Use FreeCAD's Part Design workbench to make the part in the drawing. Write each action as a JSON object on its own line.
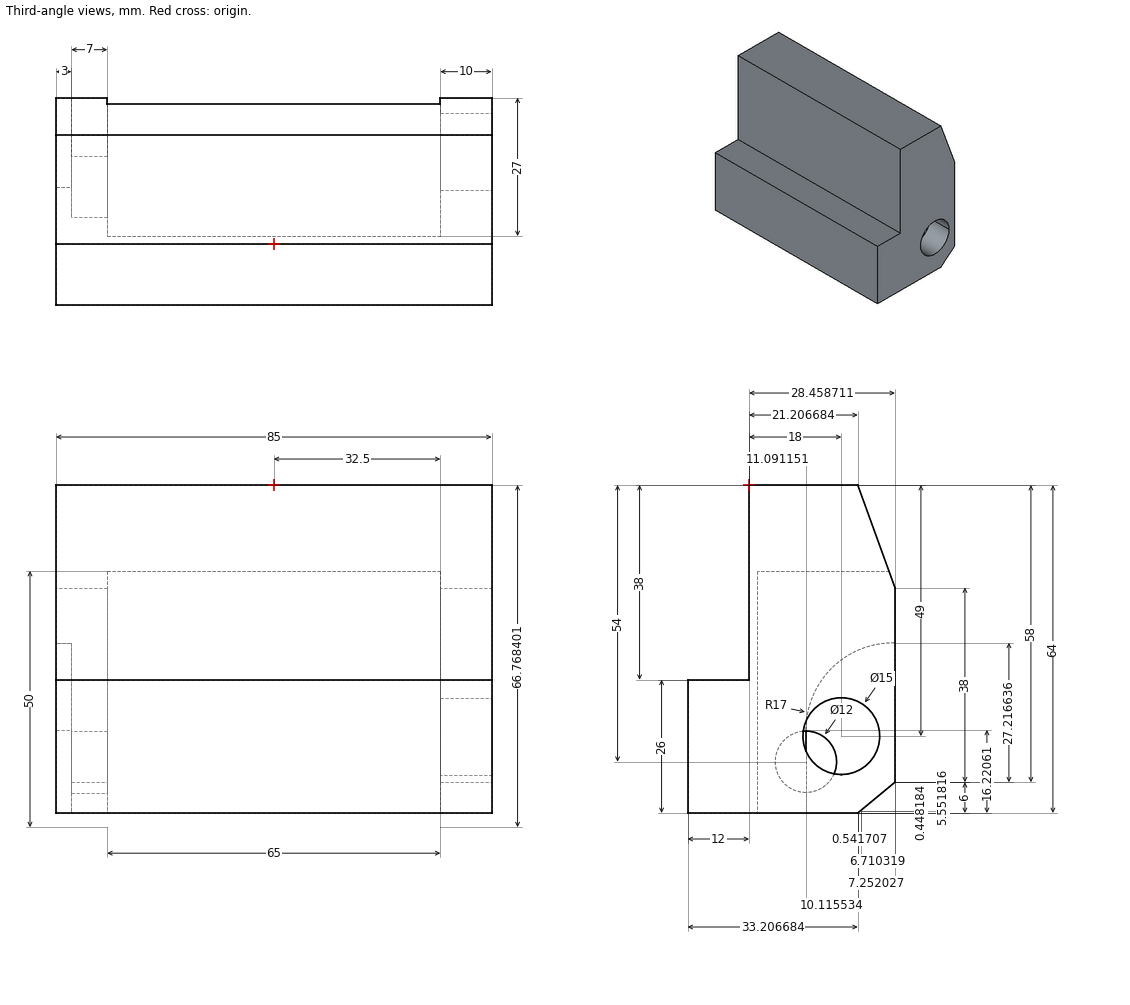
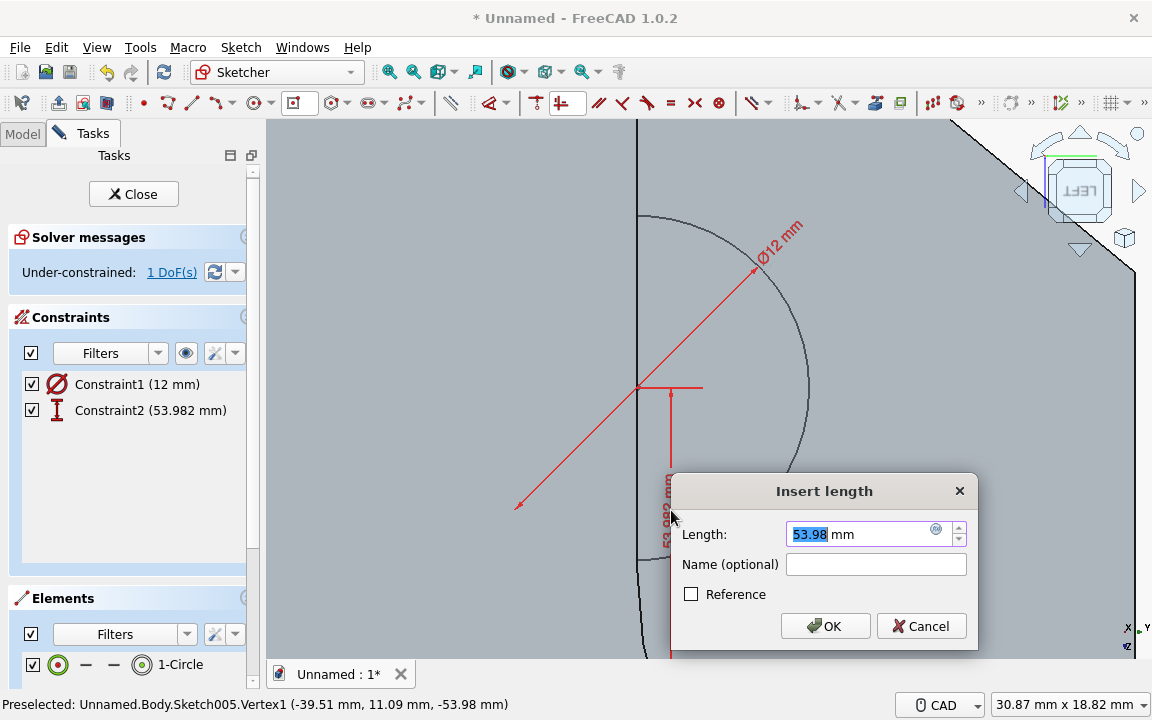
{"action": "type", "text": "54"}
{"action": "key", "text": "Return"}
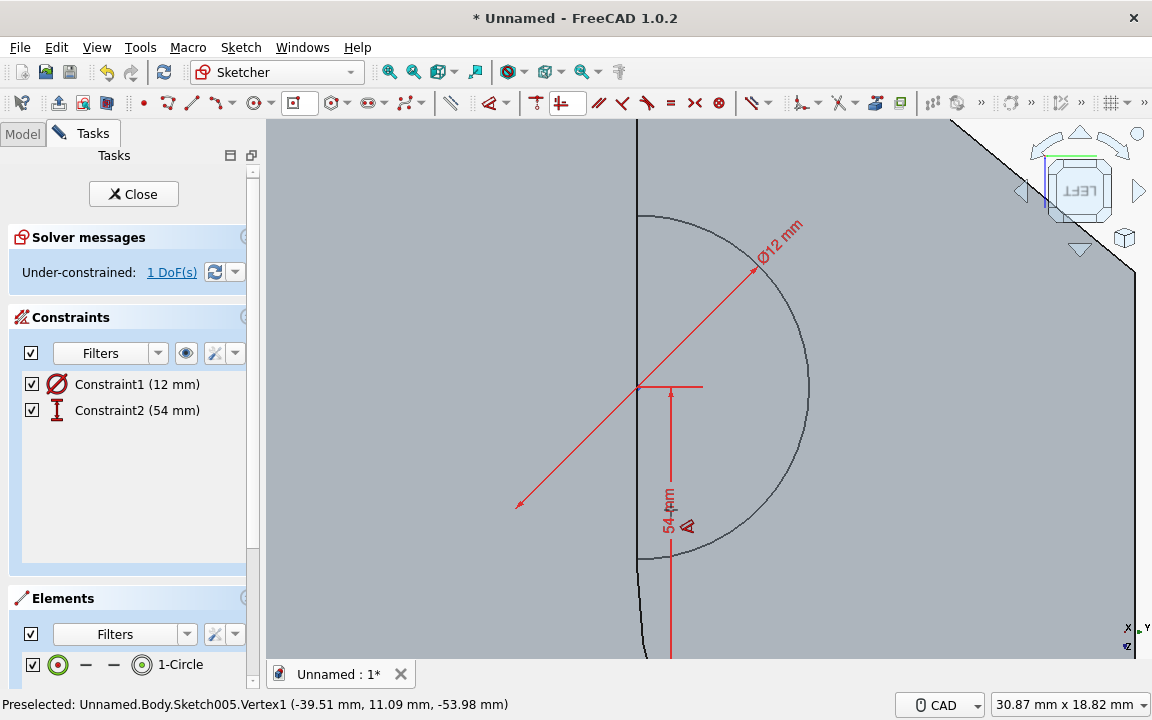
{"action": "left_click", "coordinate": [637, 387]}
{"action": "left_click", "coordinate": [405, 353]}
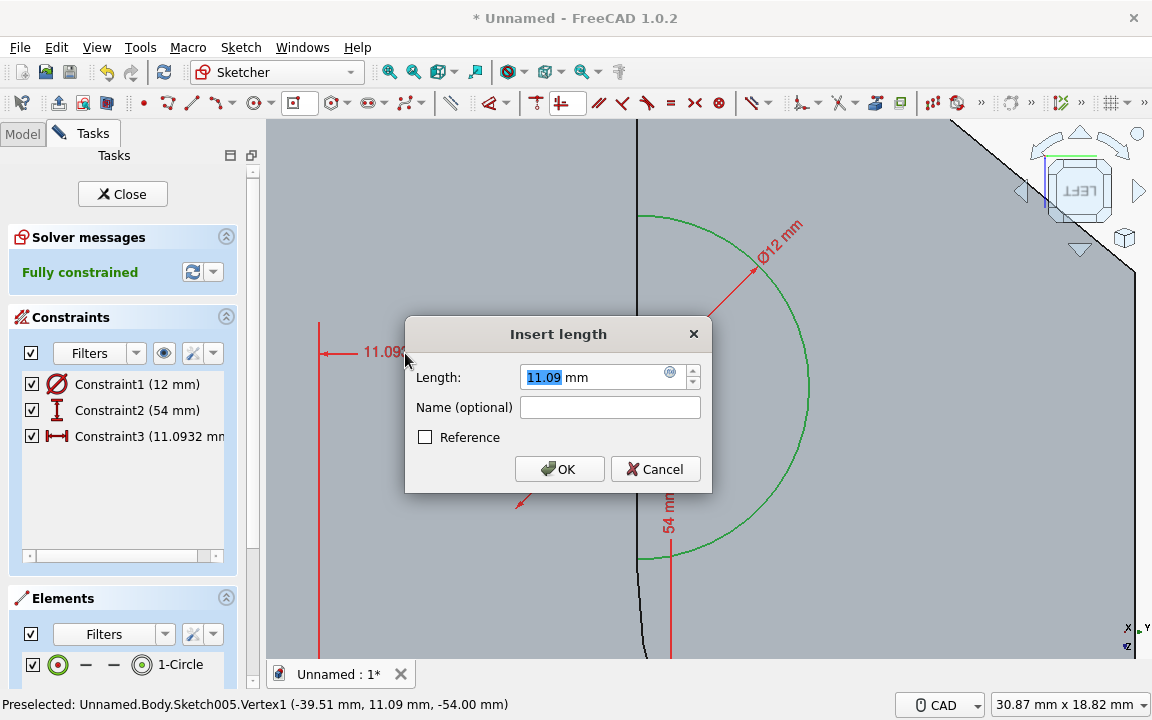
{"action": "type", "text": "11.091151"}
{"action": "key", "text": "Return"}
{"action": "key", "text": "Escape"}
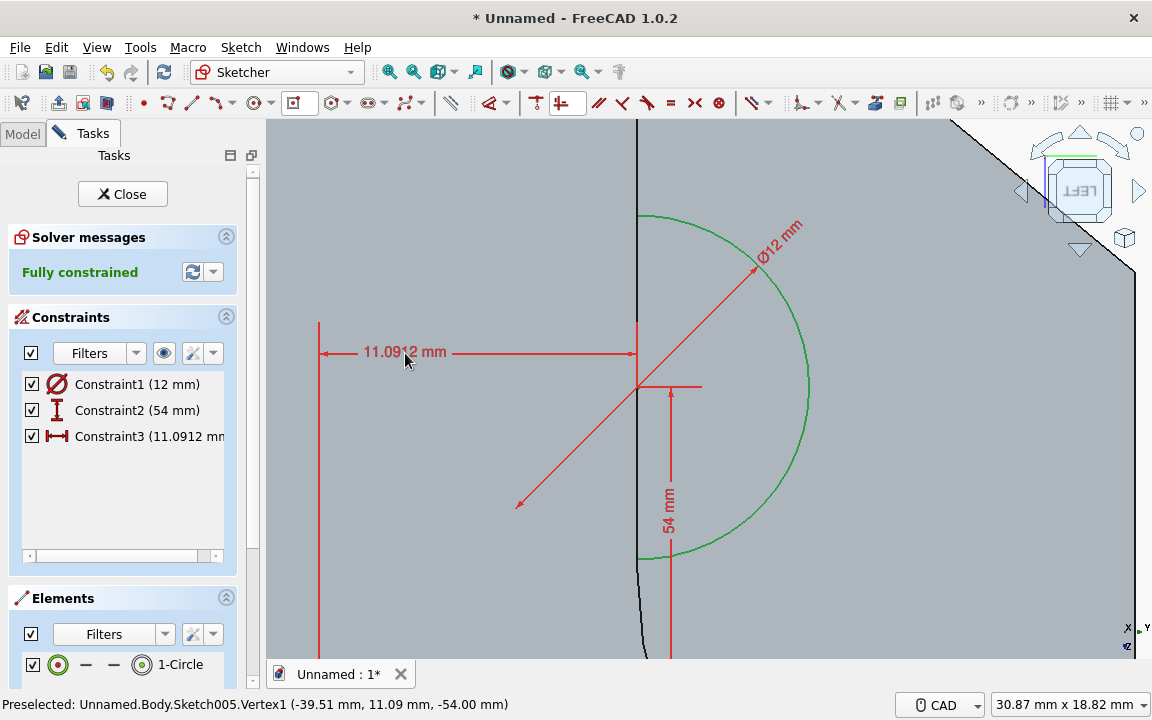
{"action": "left_click", "coordinate": [123, 194]}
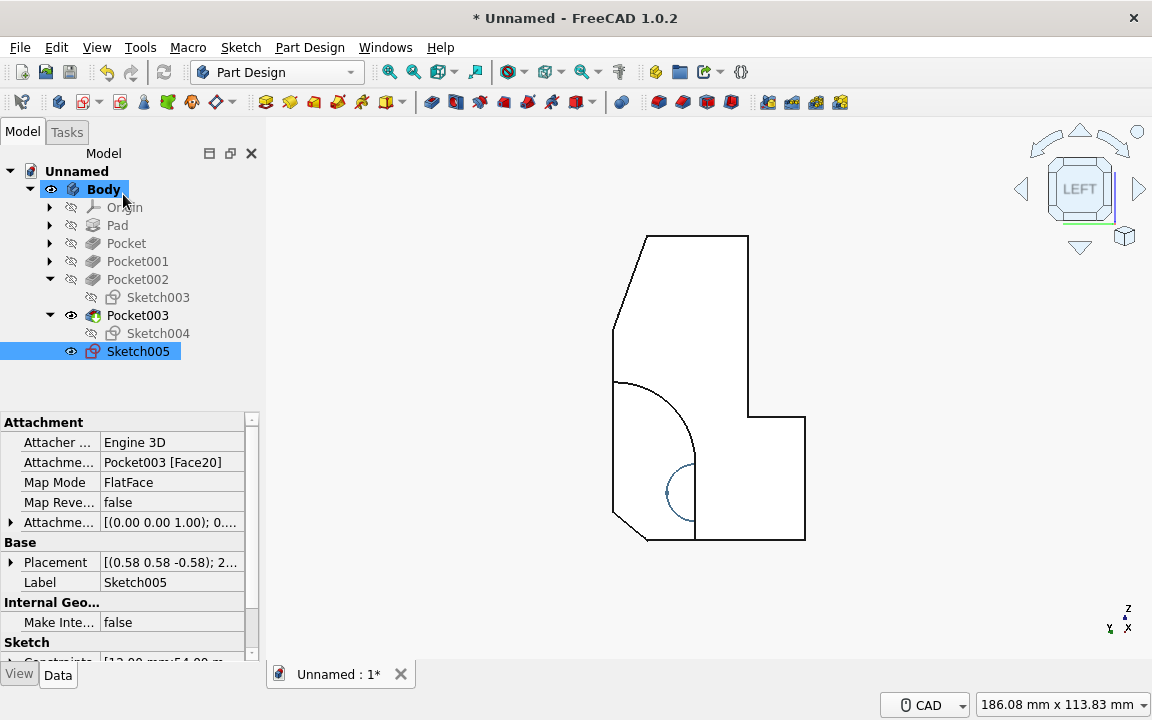
{"action": "left_click", "coordinate": [432, 102]}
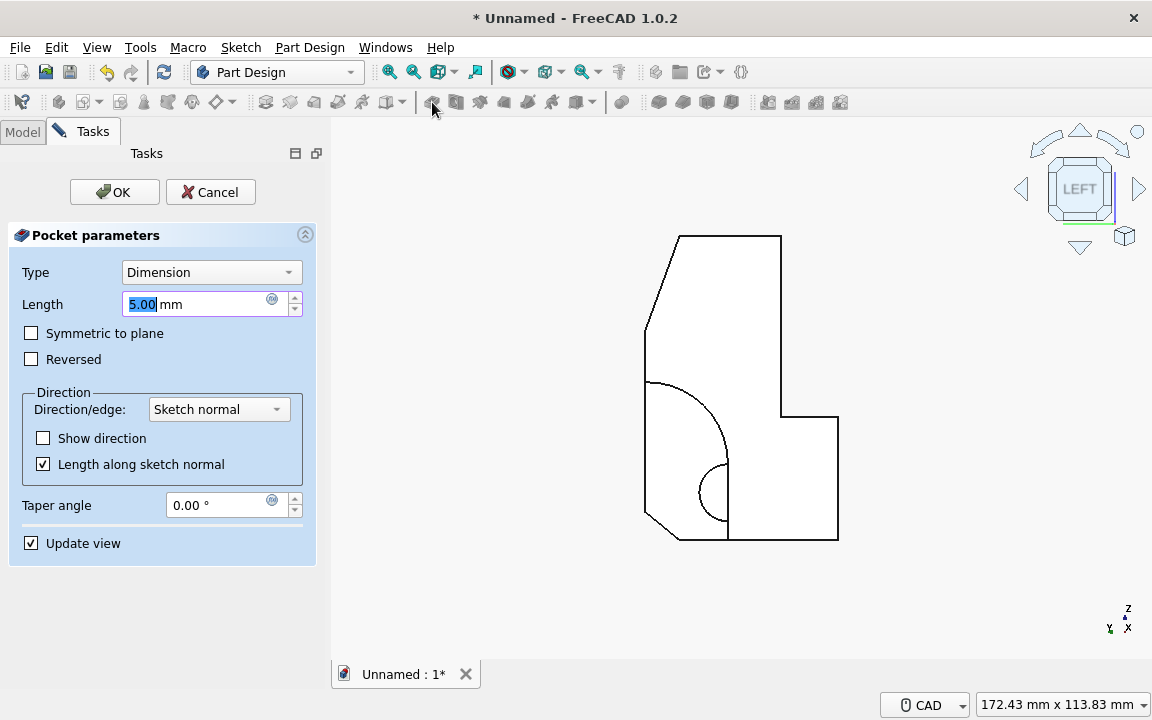
{"action": "type", "text": "7"}
{"action": "key", "text": "Tab"}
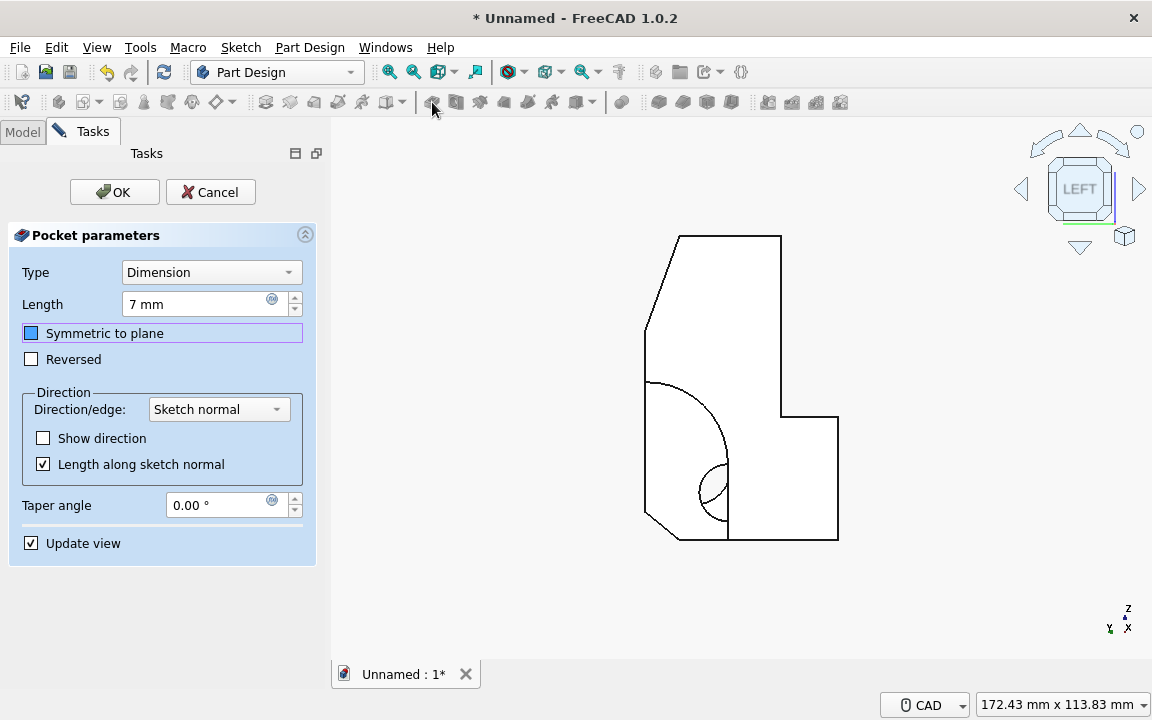
{"action": "left_click", "coordinate": [115, 192]}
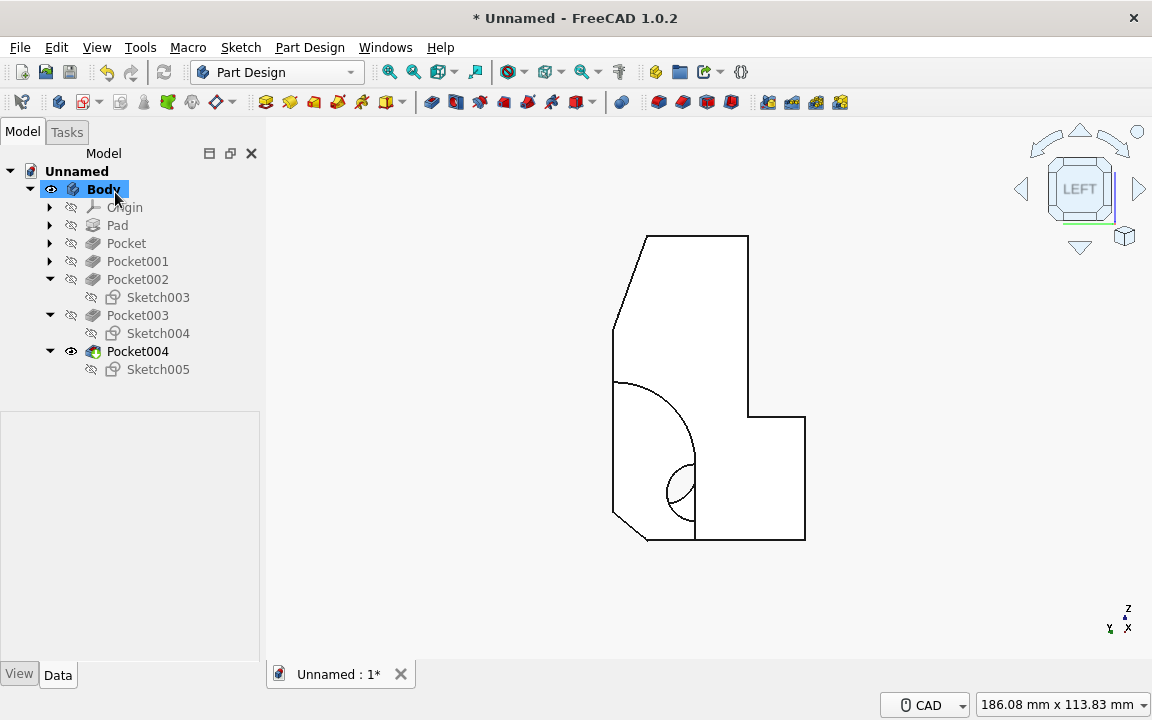
{"action": "key", "text": "0"}